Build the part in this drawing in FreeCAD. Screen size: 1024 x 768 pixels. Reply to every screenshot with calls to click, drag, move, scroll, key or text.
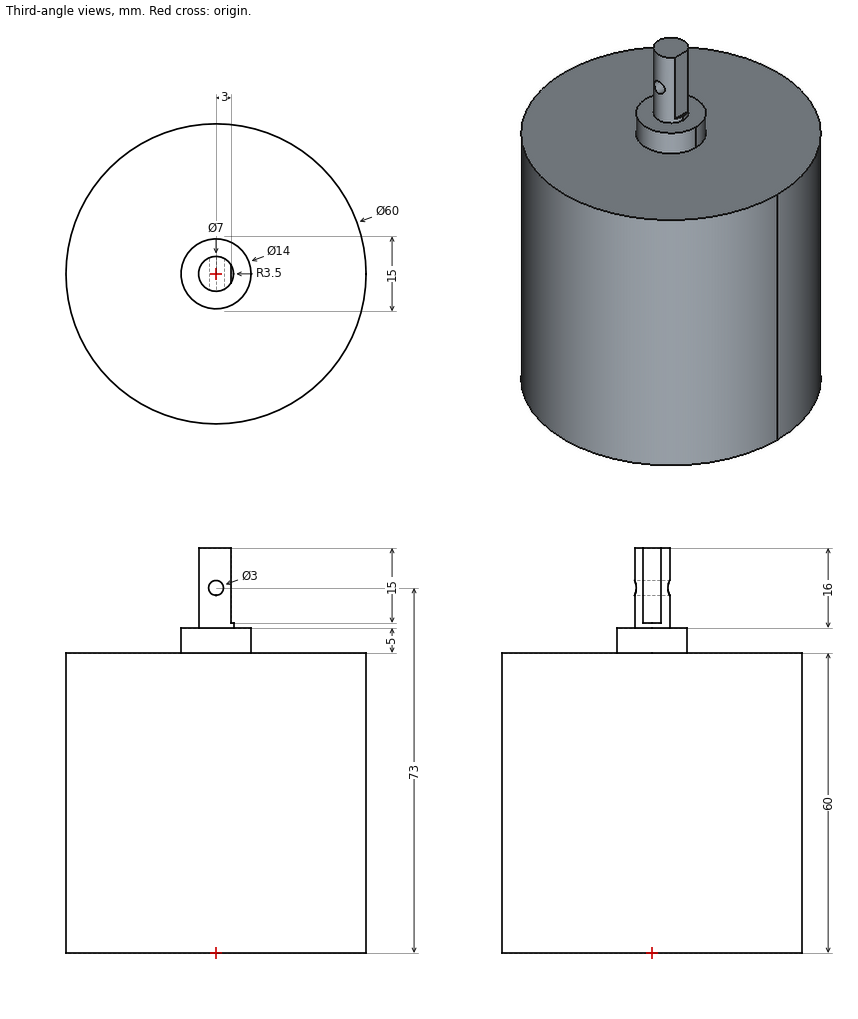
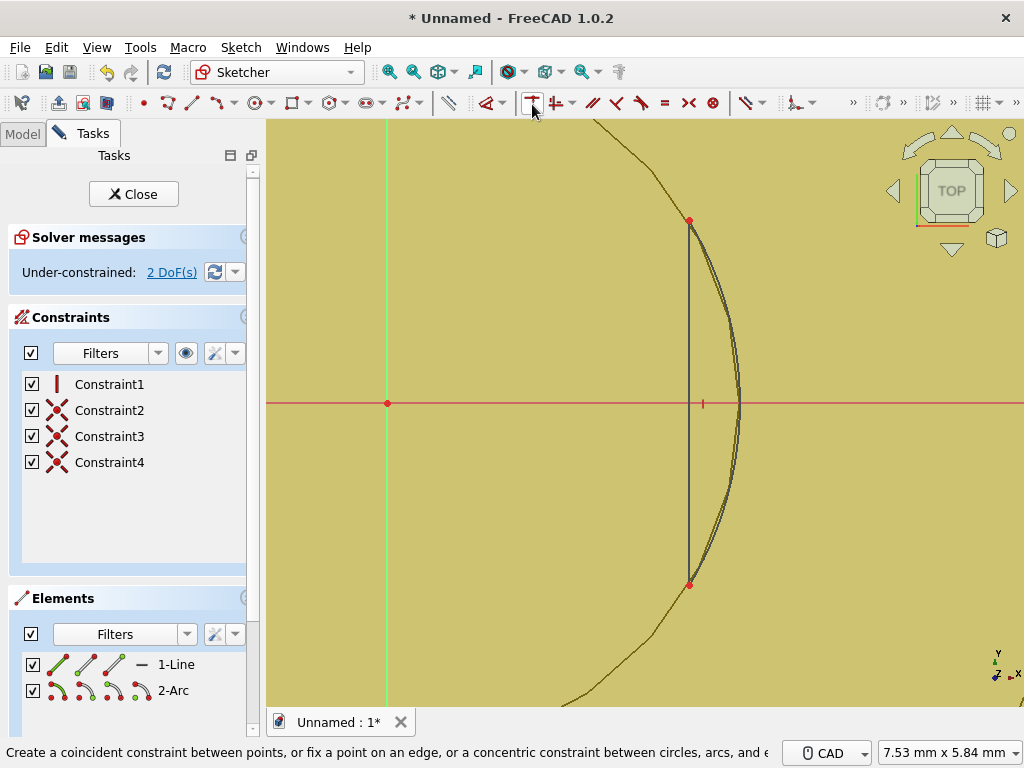
click(486, 104)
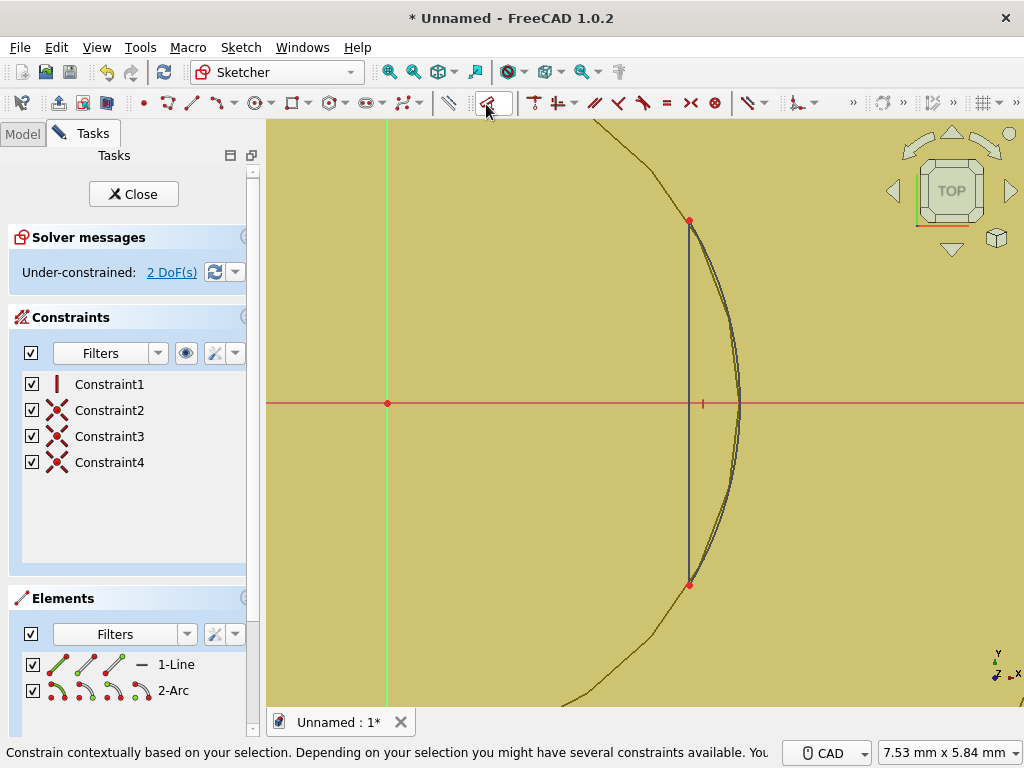
click(732, 480)
click(763, 487)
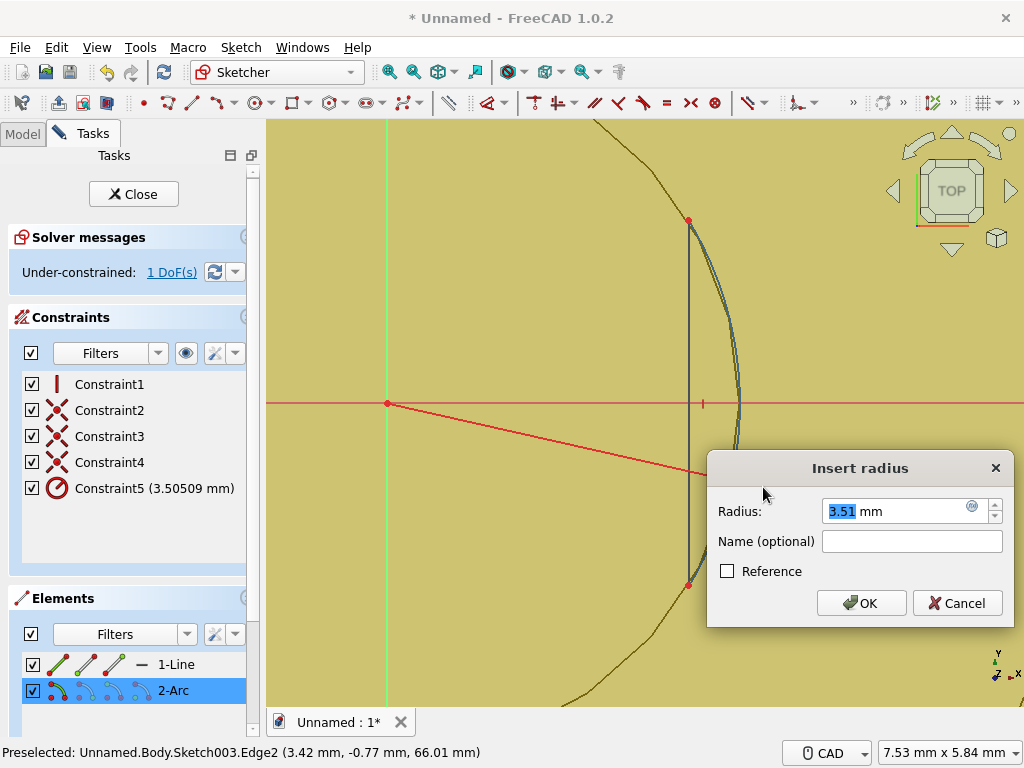
text(3.5)
key(Return)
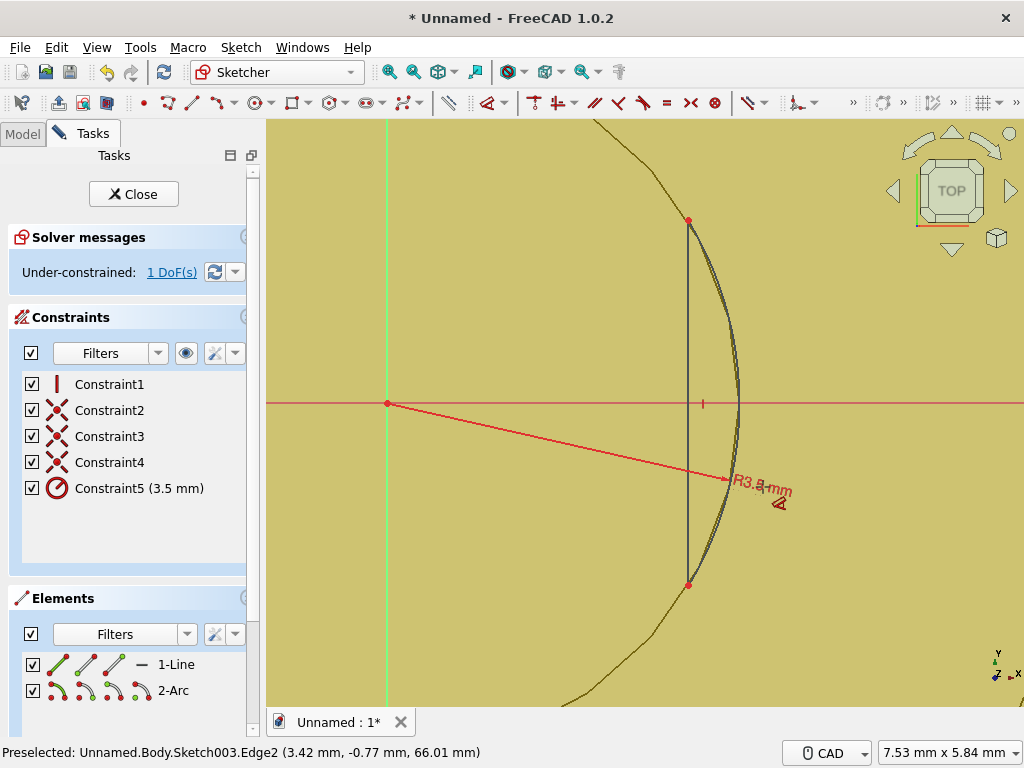
click(688, 221)
click(538, 187)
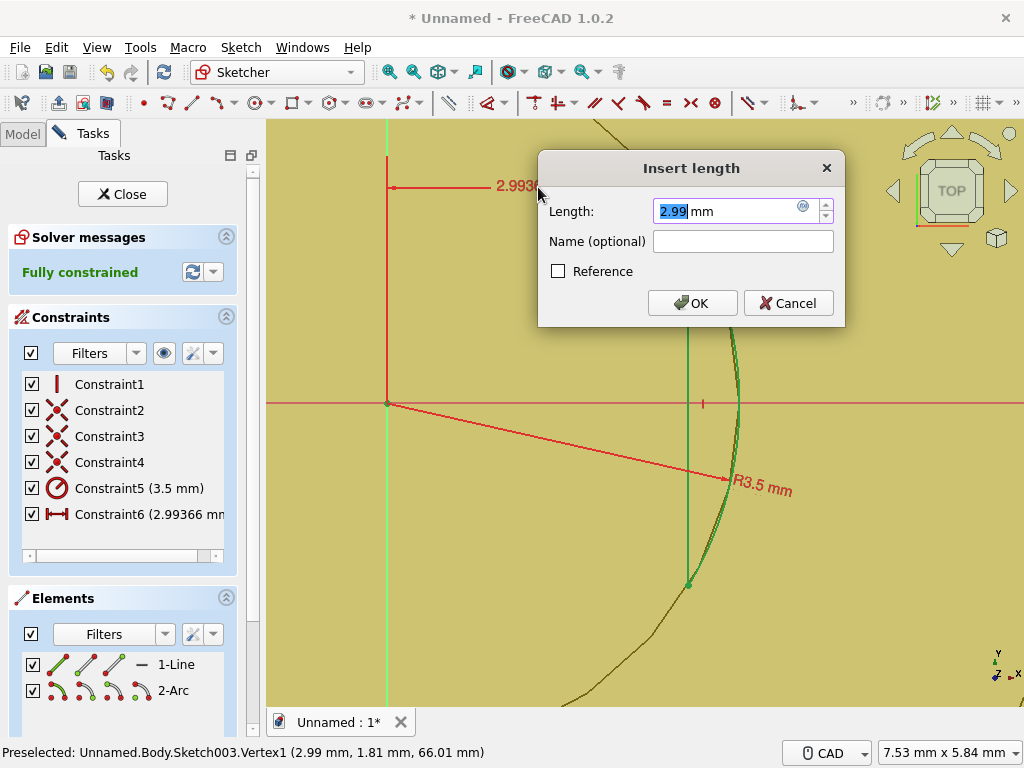
text(3)
key(Return)
key(Escape)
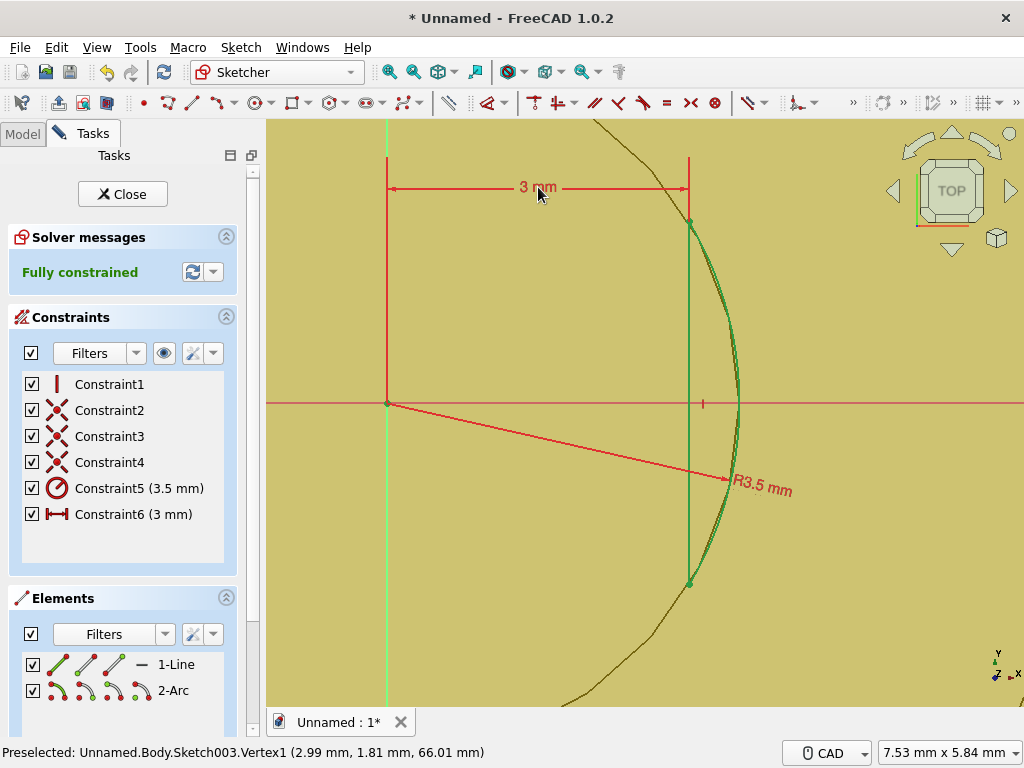
click(123, 194)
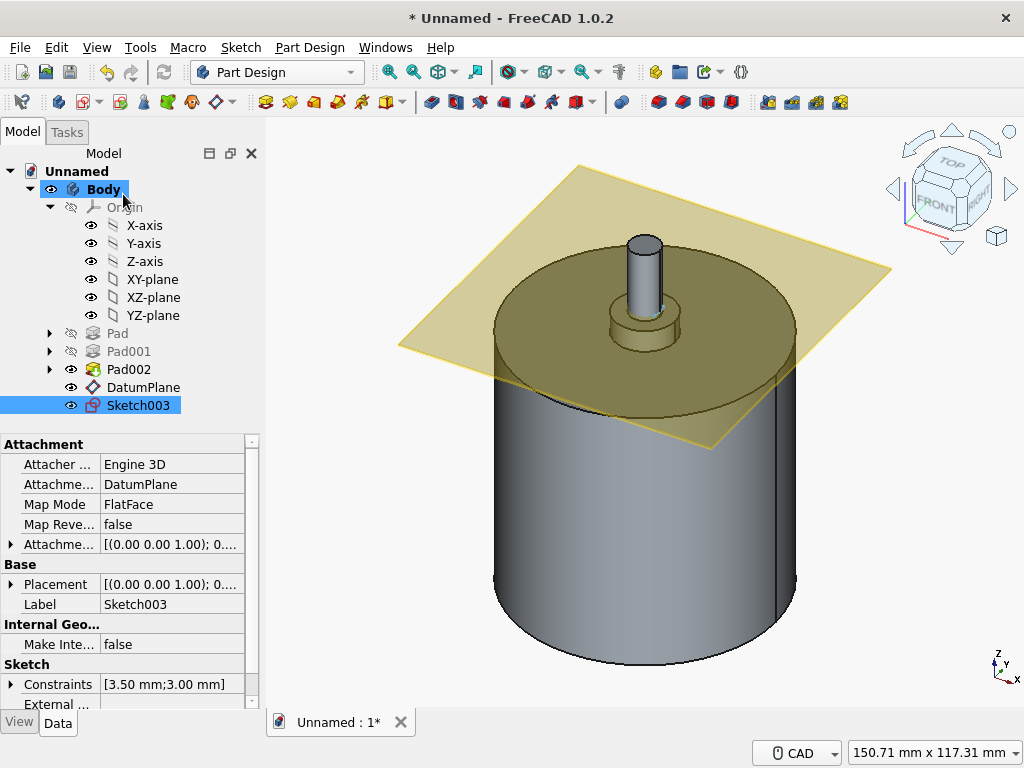
click(432, 102)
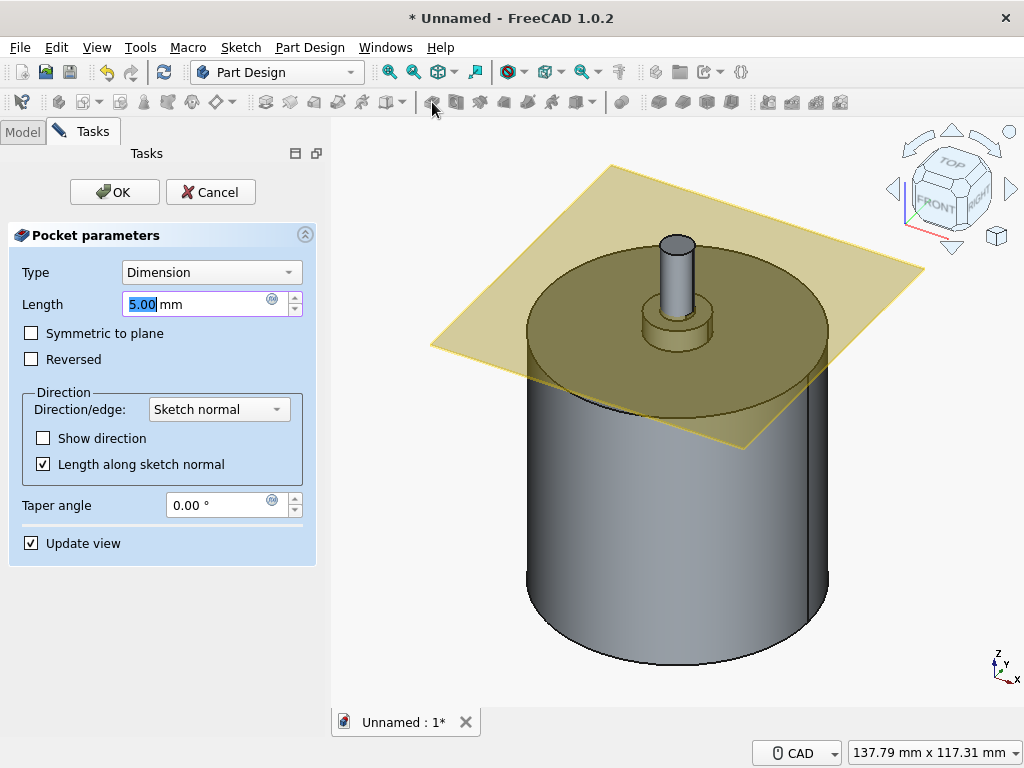
text(15)
key(Tab)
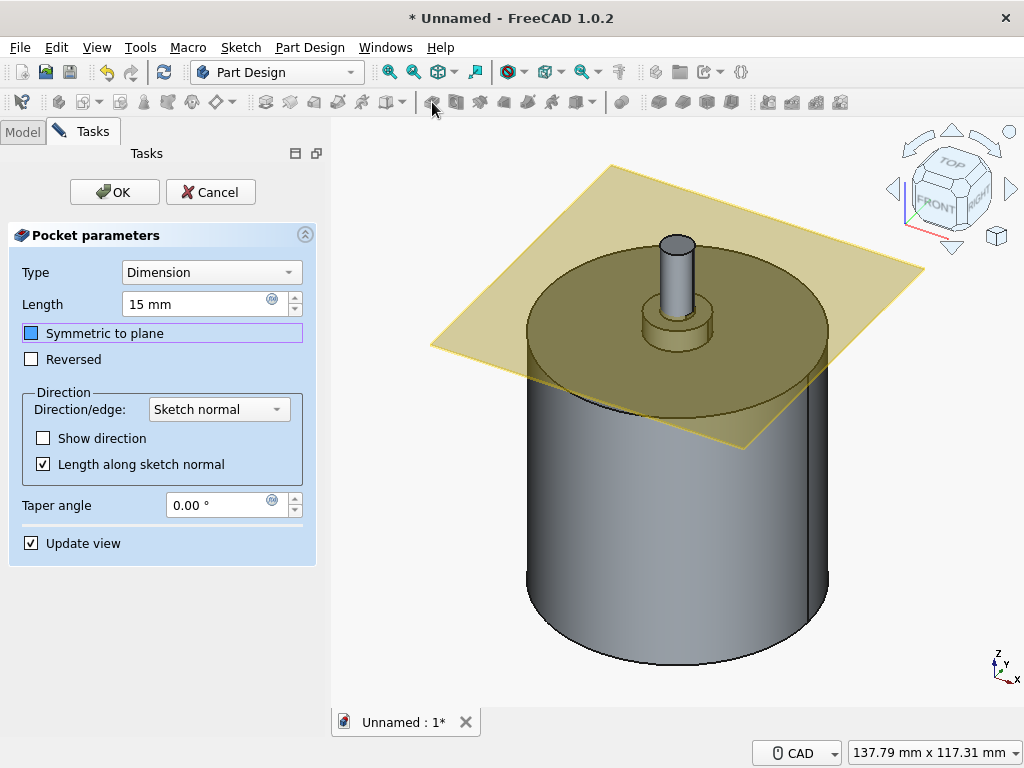
click(30, 359)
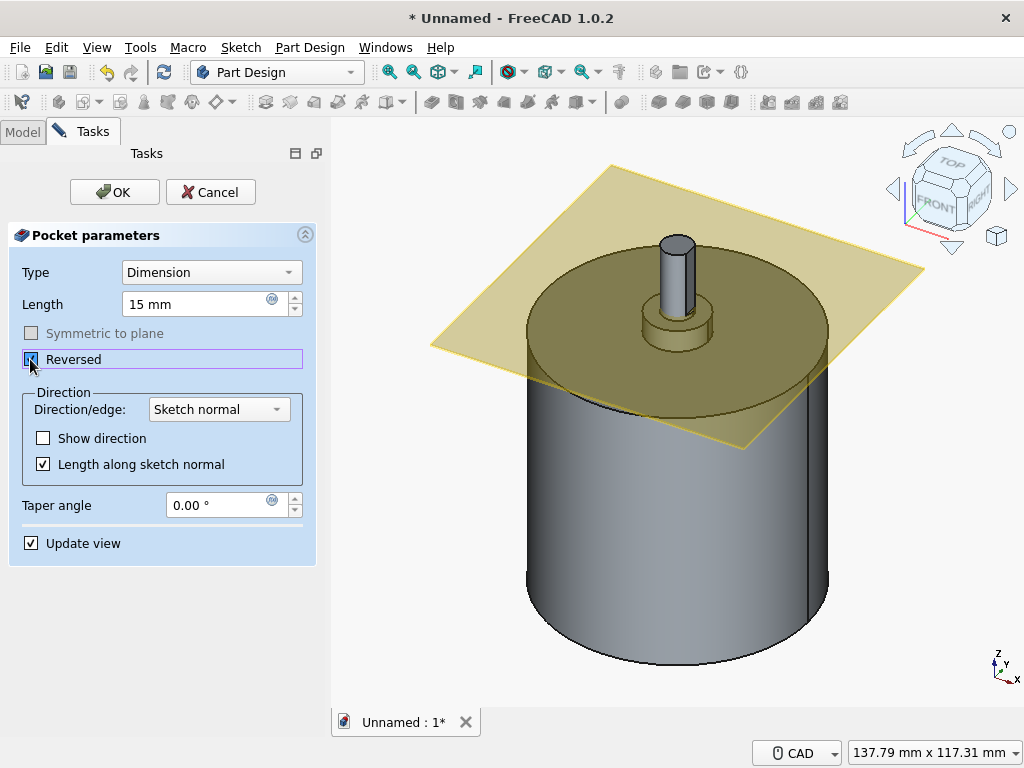
click(115, 192)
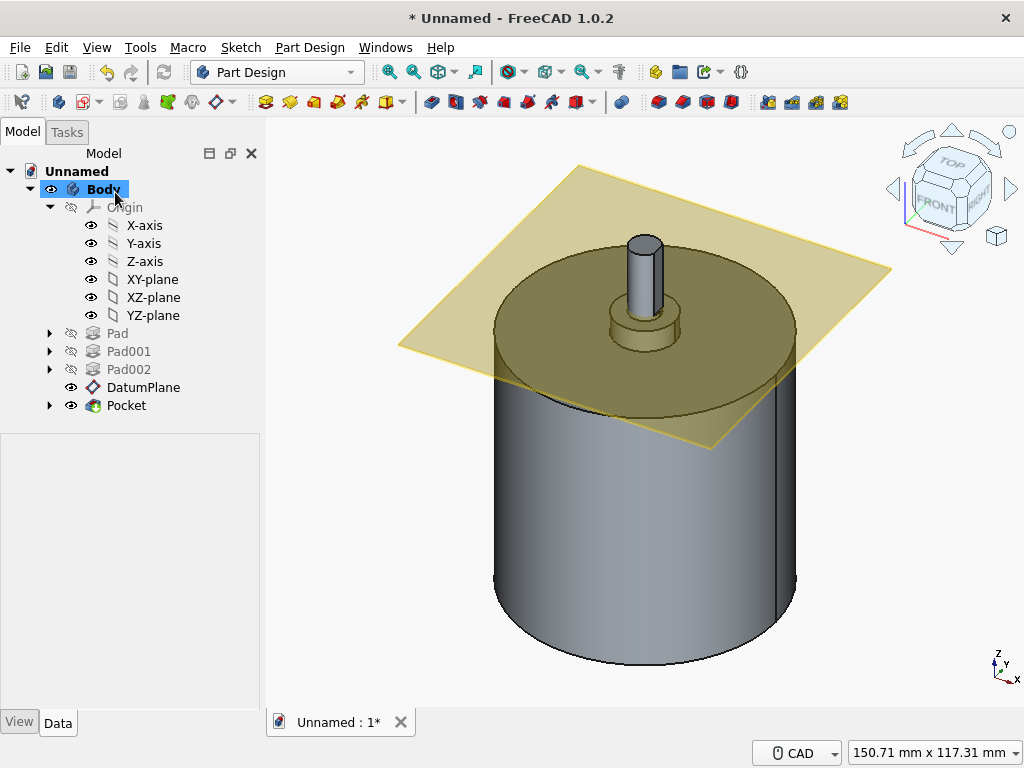
click(116, 387)
key(space)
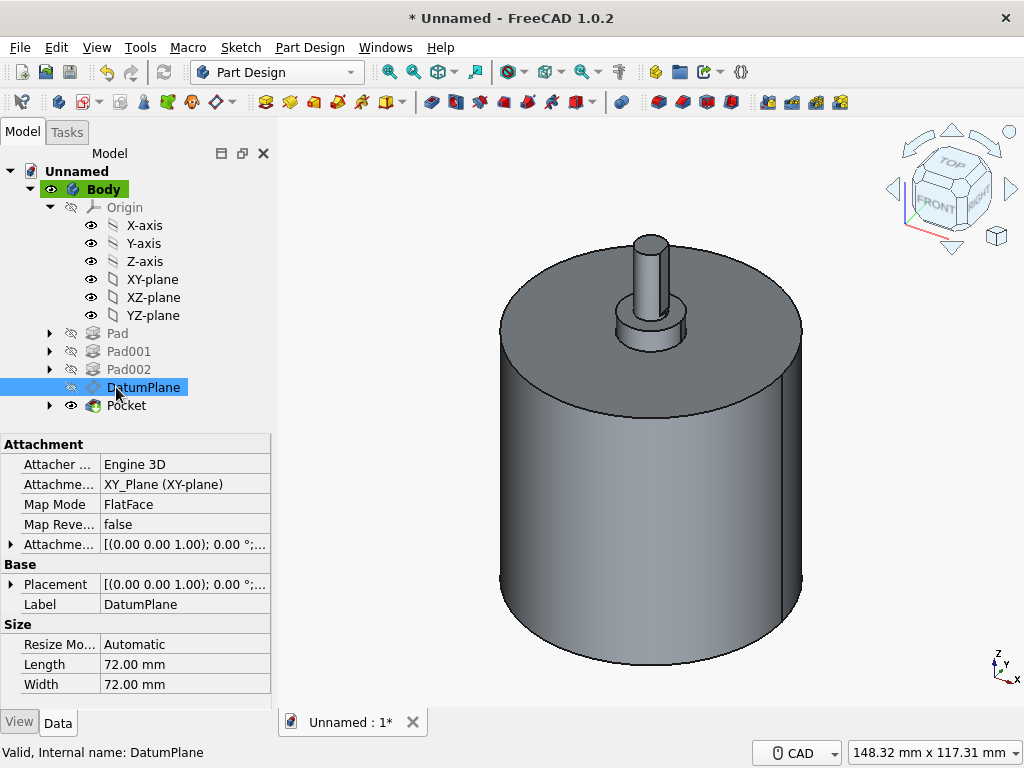
click(318, 667)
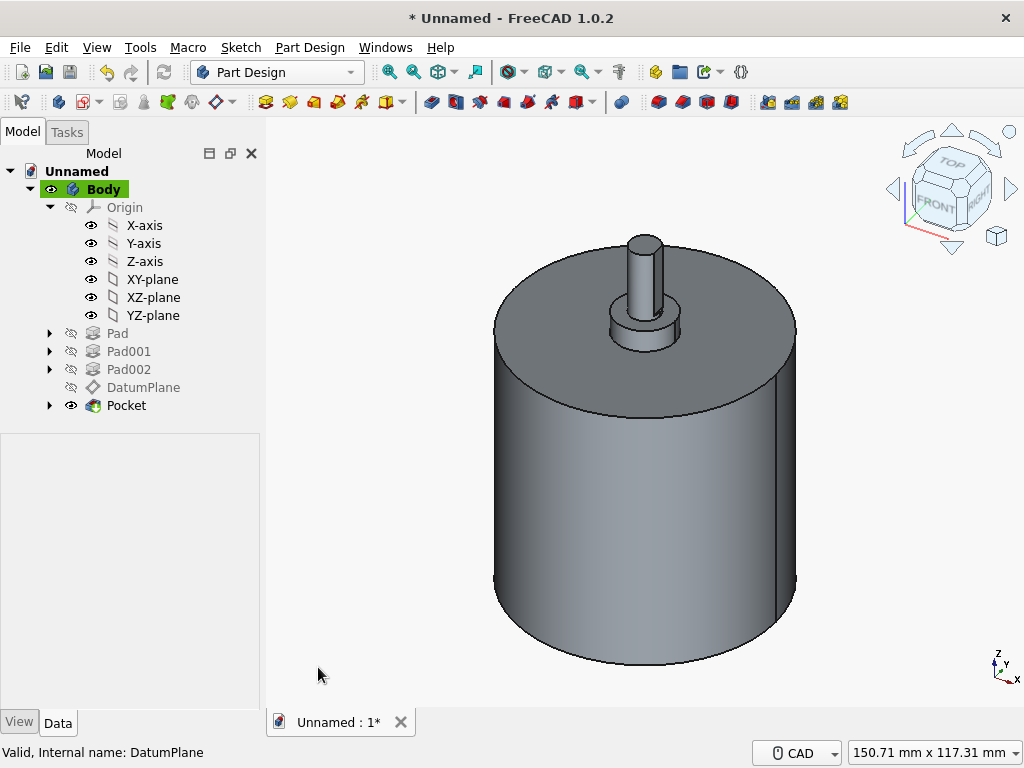
click(84, 102)